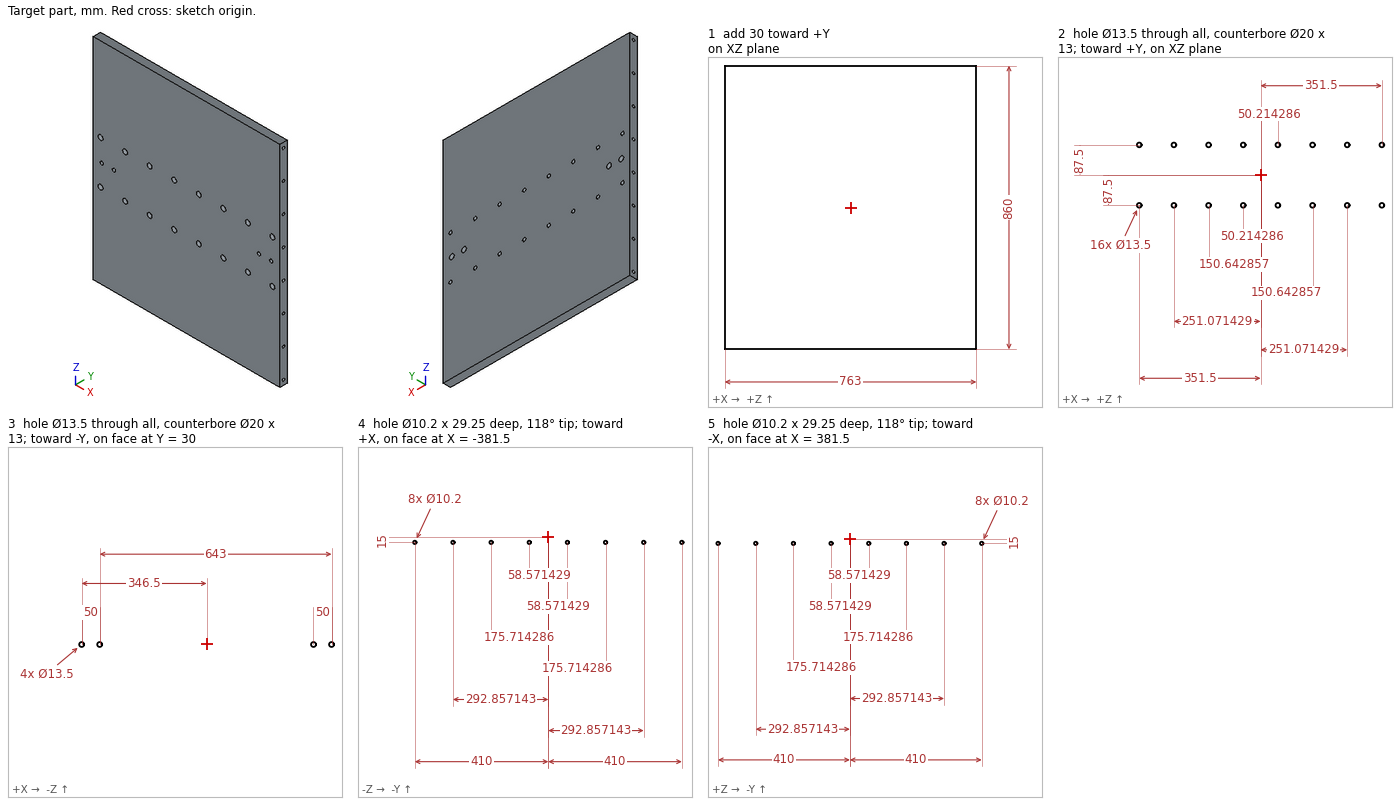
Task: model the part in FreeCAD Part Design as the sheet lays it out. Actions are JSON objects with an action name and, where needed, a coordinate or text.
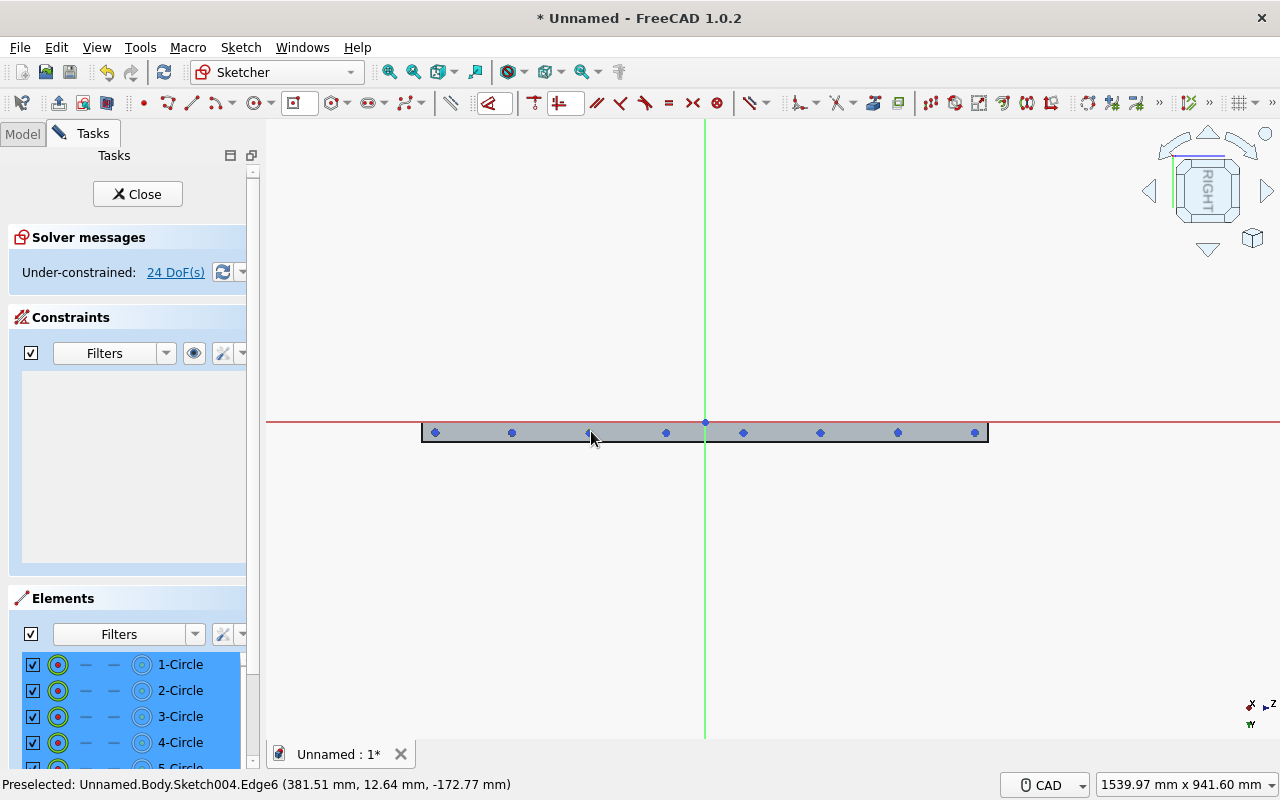
{"action": "scroll", "coordinate": [514, 431], "scroll_direction": "up", "scroll_amount": 8}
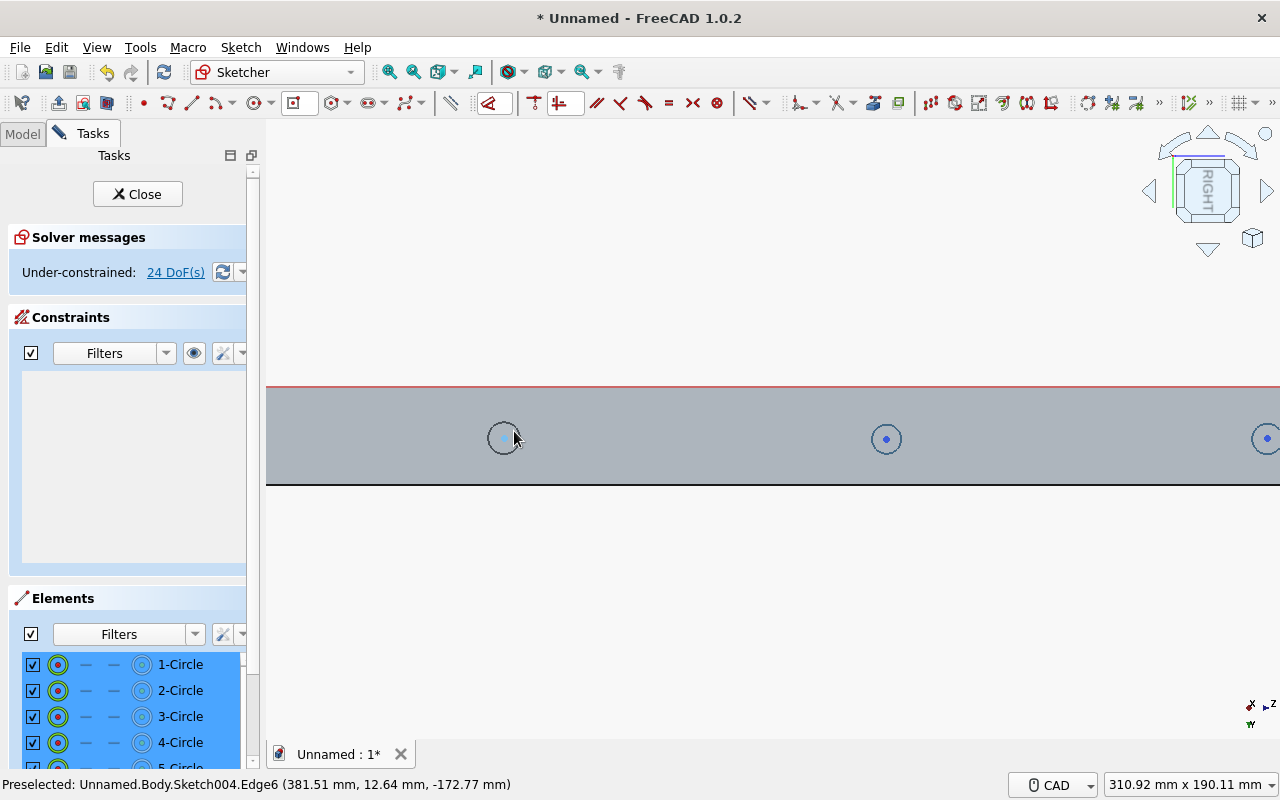
{"action": "left_click", "coordinate": [515, 427]}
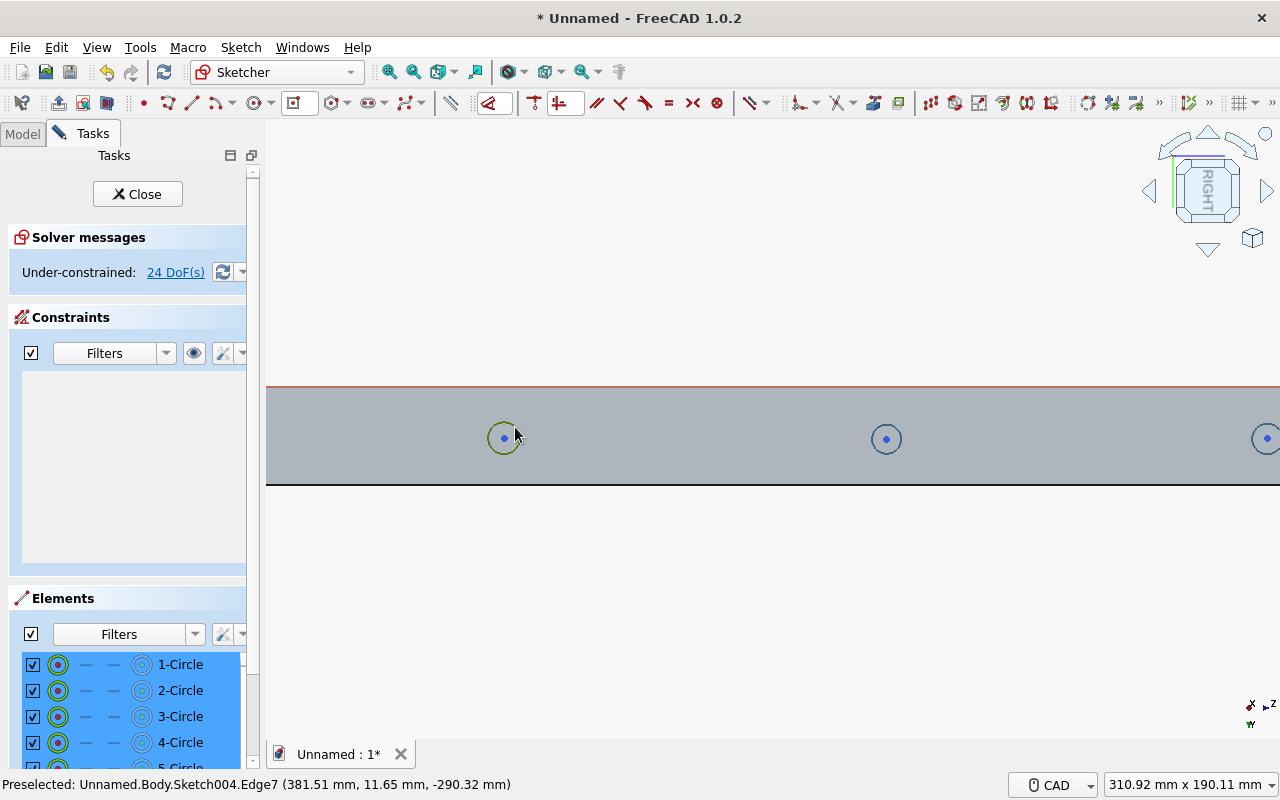
{"action": "scroll", "coordinate": [514, 431], "scroll_direction": "down", "scroll_amount": 8}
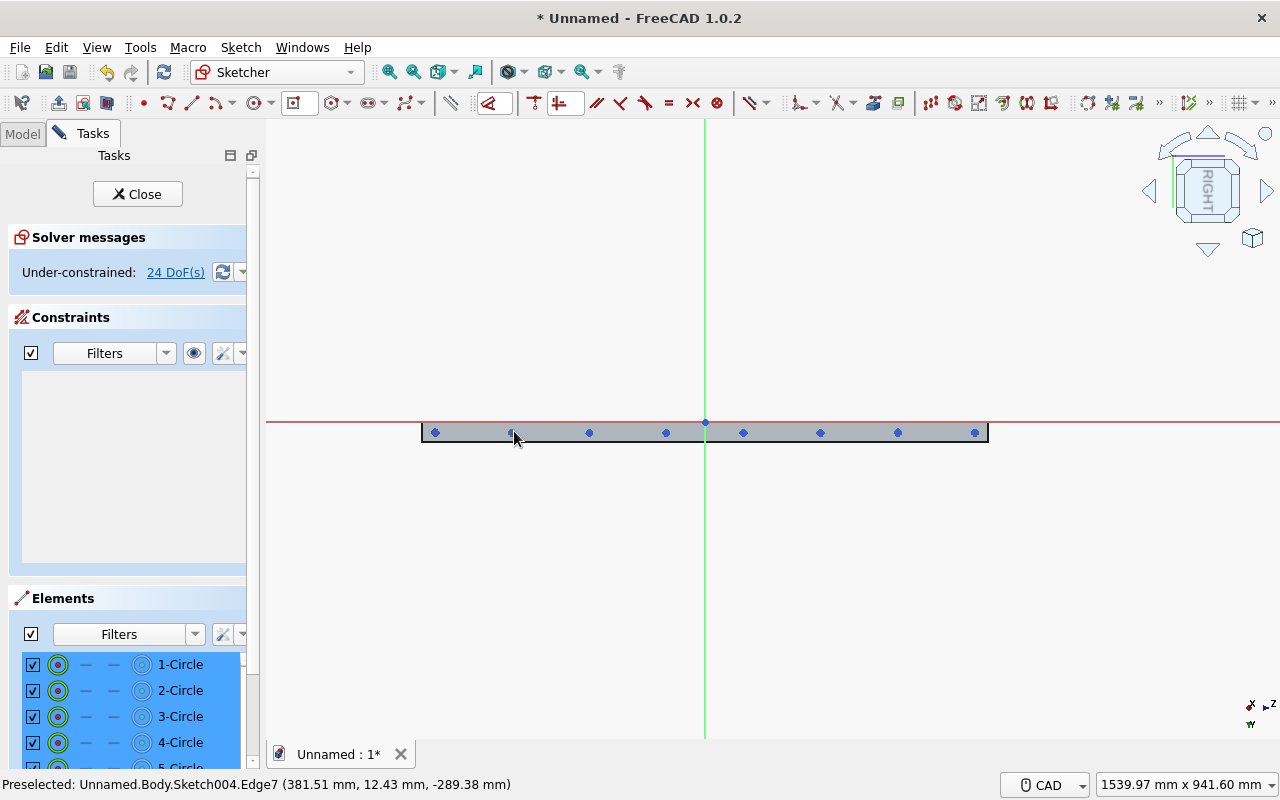
{"action": "scroll", "coordinate": [438, 430], "scroll_direction": "up", "scroll_amount": 8}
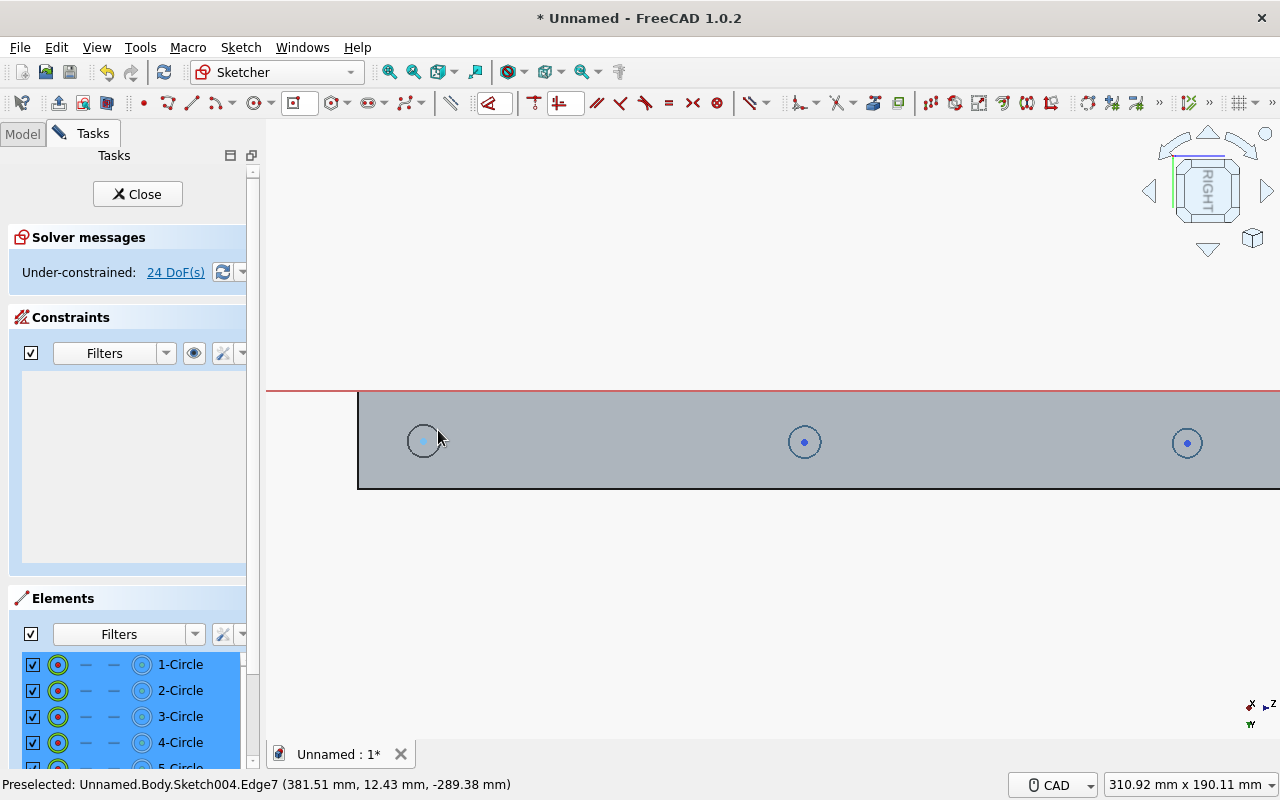
{"action": "left_click", "coordinate": [435, 430]}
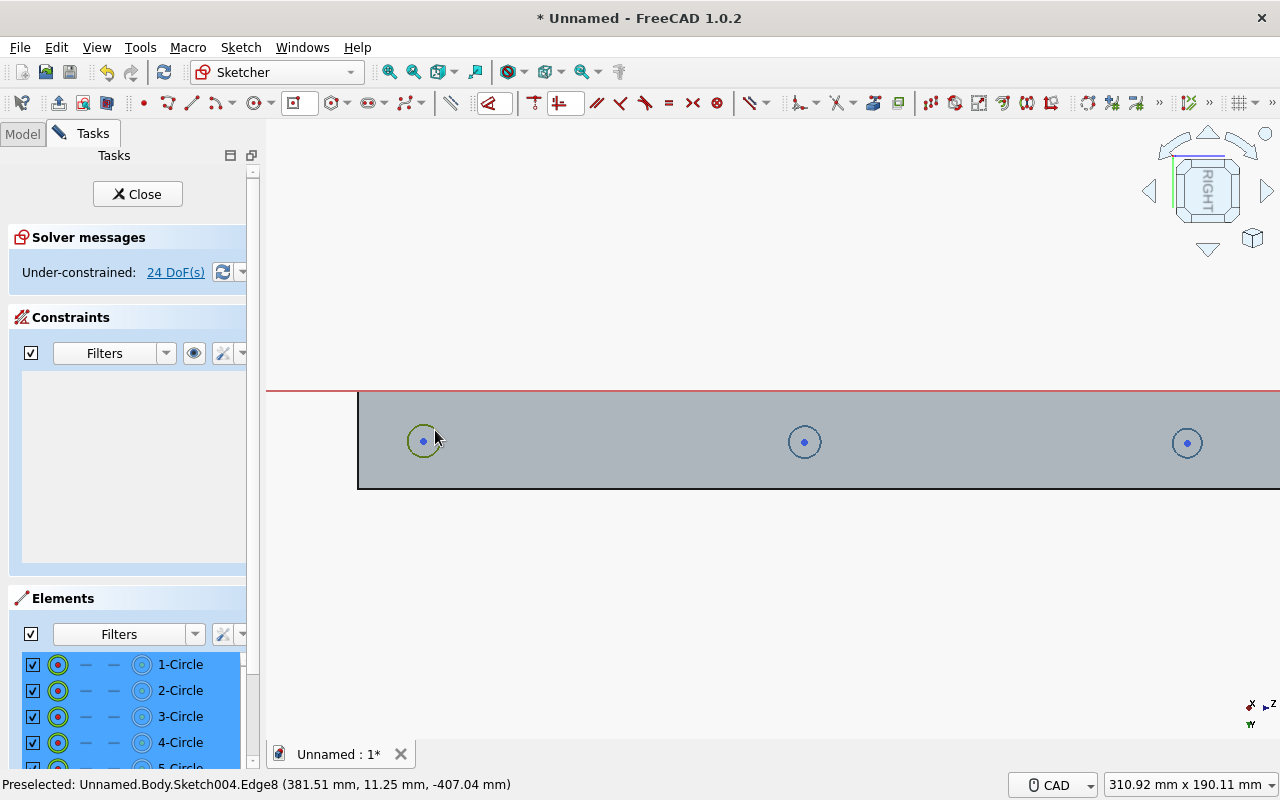
{"action": "left_click", "coordinate": [670, 104]}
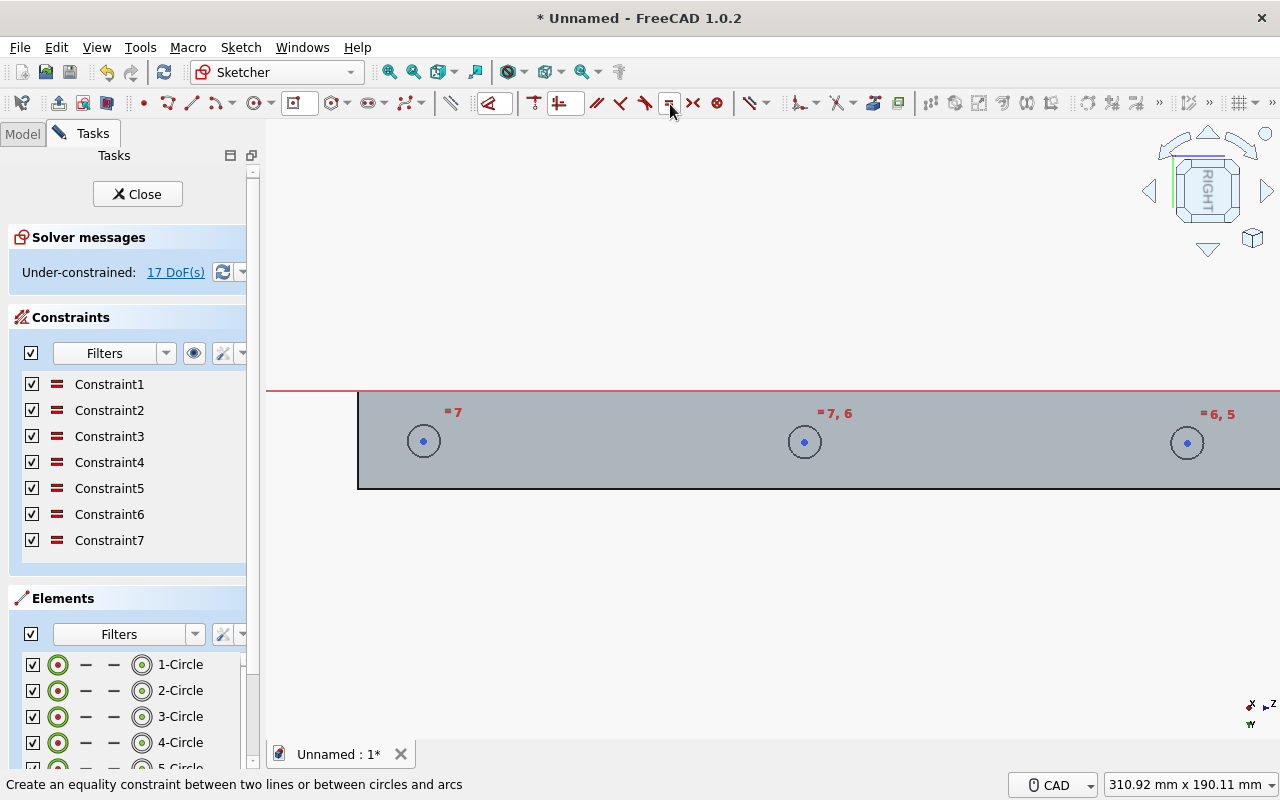
{"action": "scroll", "coordinate": [437, 430], "scroll_direction": "down", "scroll_amount": 8}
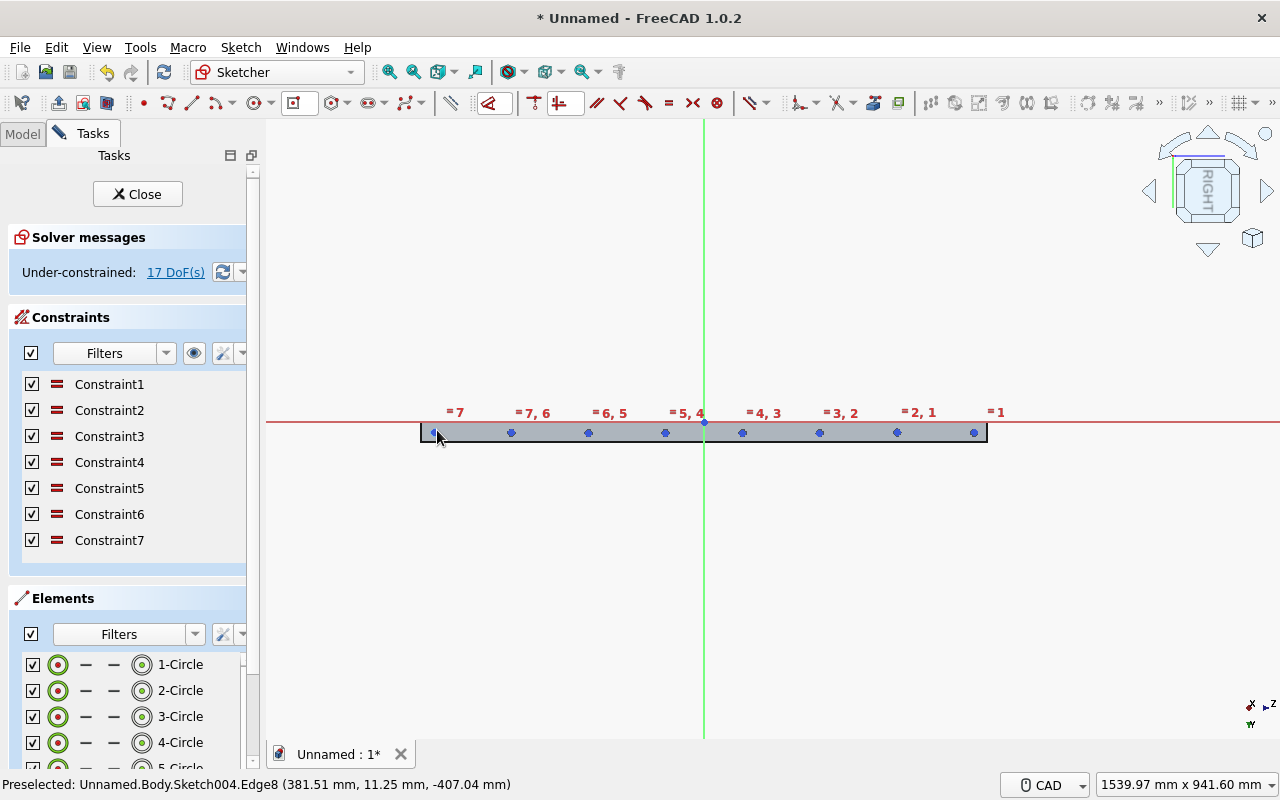
{"action": "left_click", "coordinate": [974, 433]}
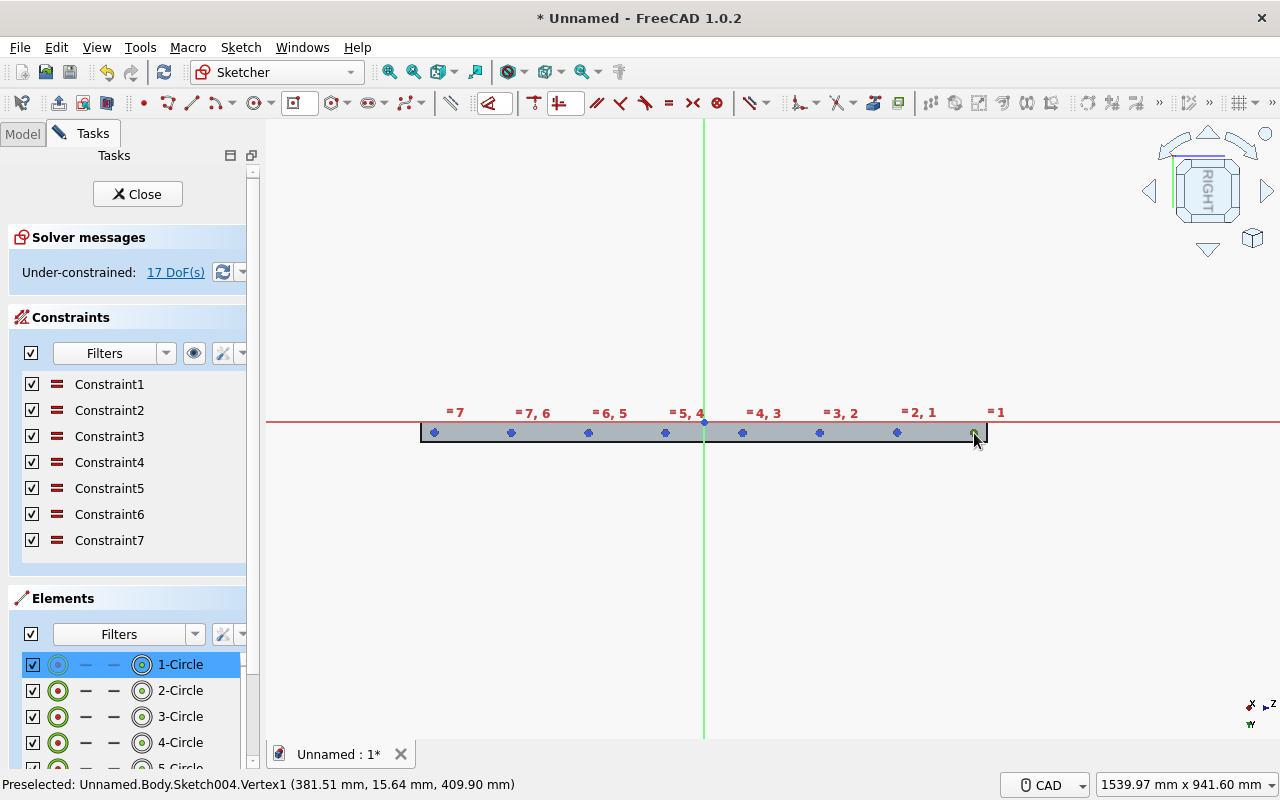
{"action": "left_click", "coordinate": [897, 433]}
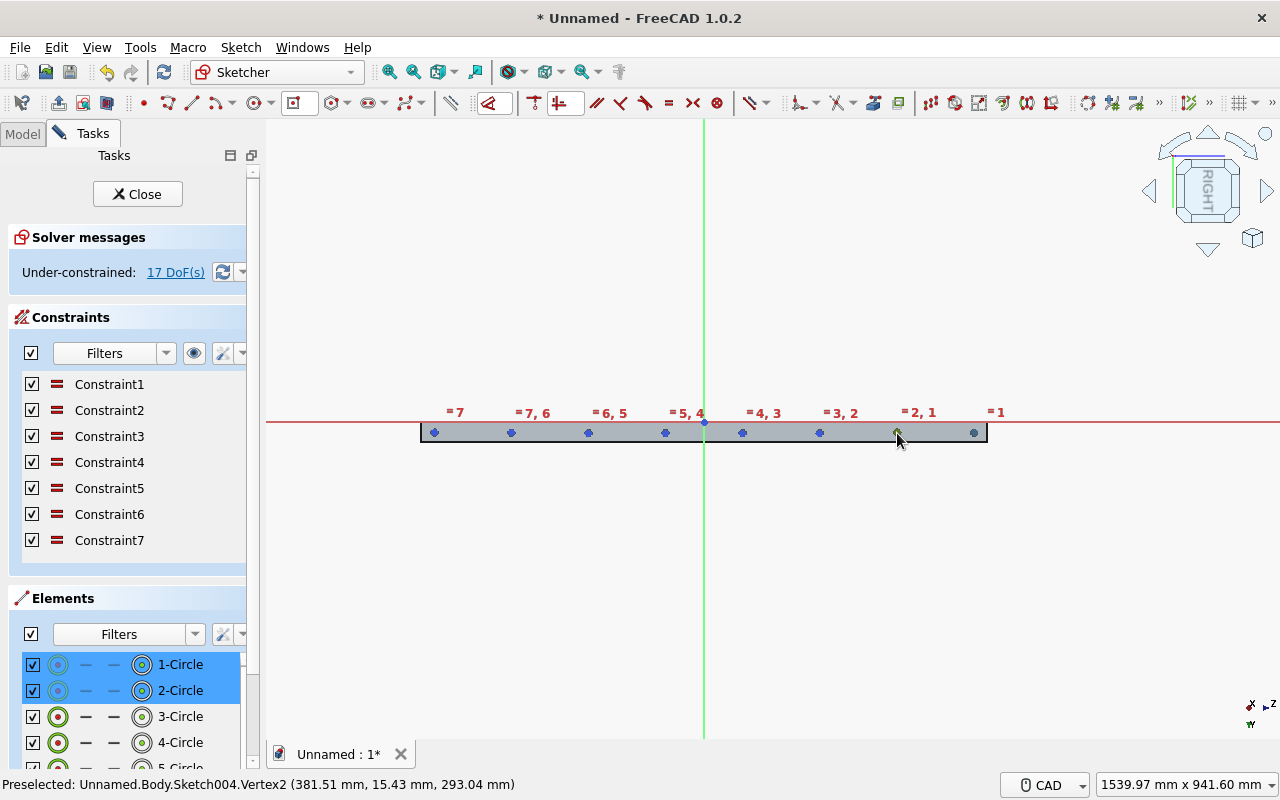
{"action": "left_click", "coordinate": [578, 104]}